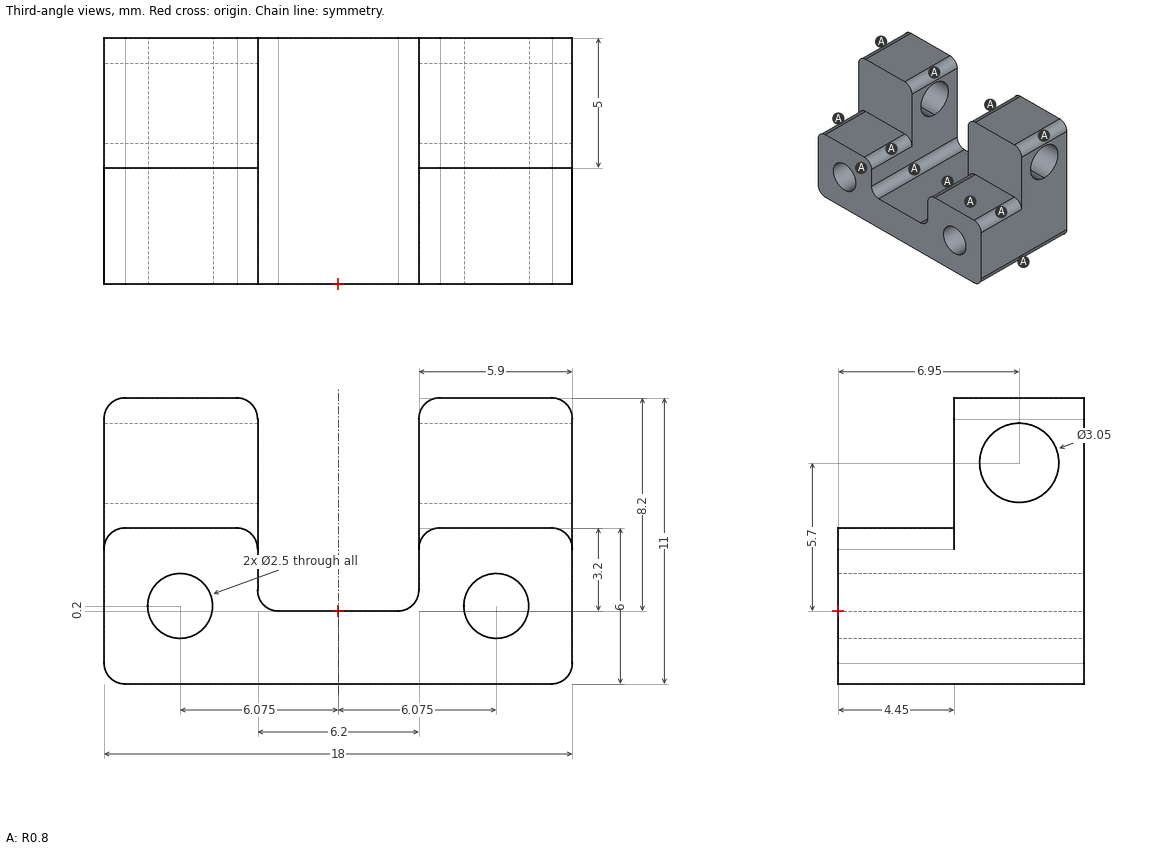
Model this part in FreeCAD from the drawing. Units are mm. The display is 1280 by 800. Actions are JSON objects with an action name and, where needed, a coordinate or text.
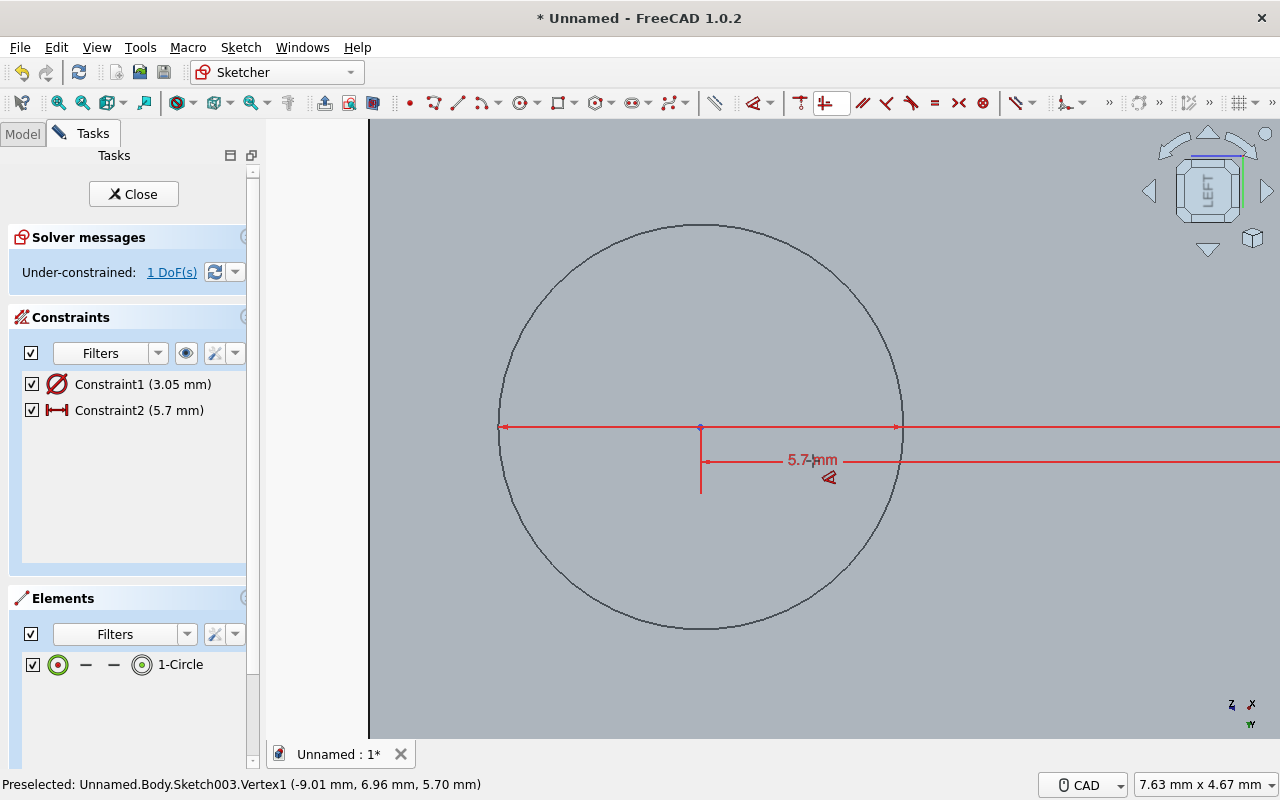
{"action": "left_click", "coordinate": [701, 427]}
{"action": "left_click", "coordinate": [667, 287]}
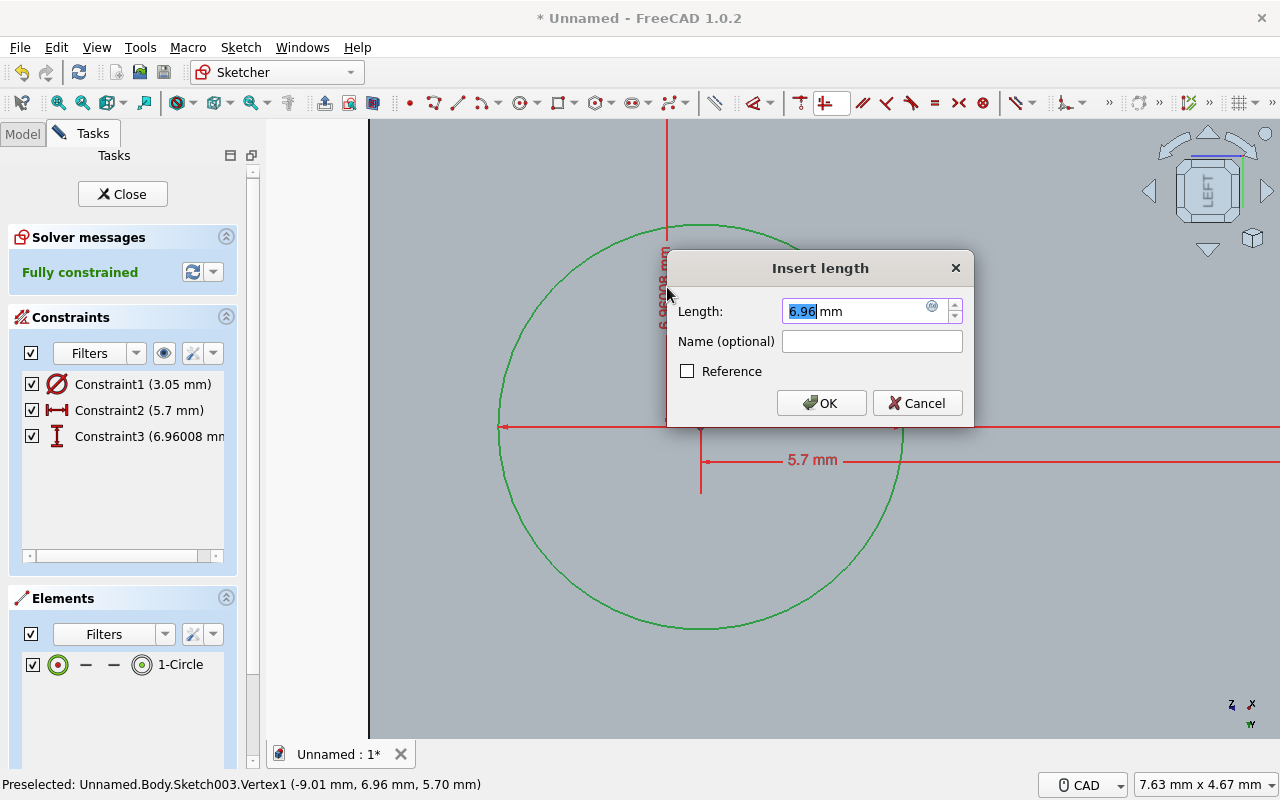
{"action": "type", "text": "6.95"}
{"action": "key", "text": "Return"}
{"action": "key", "text": "Escape"}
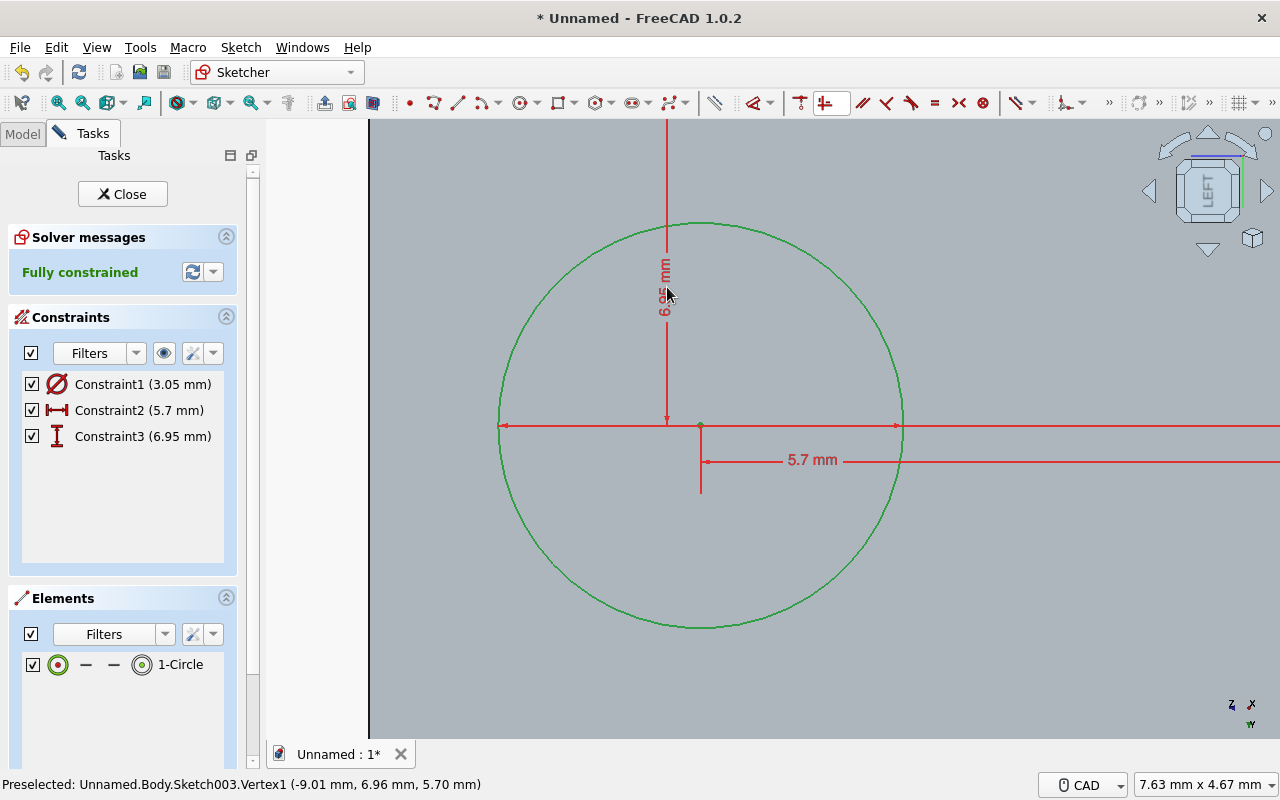
{"action": "left_click", "coordinate": [123, 194]}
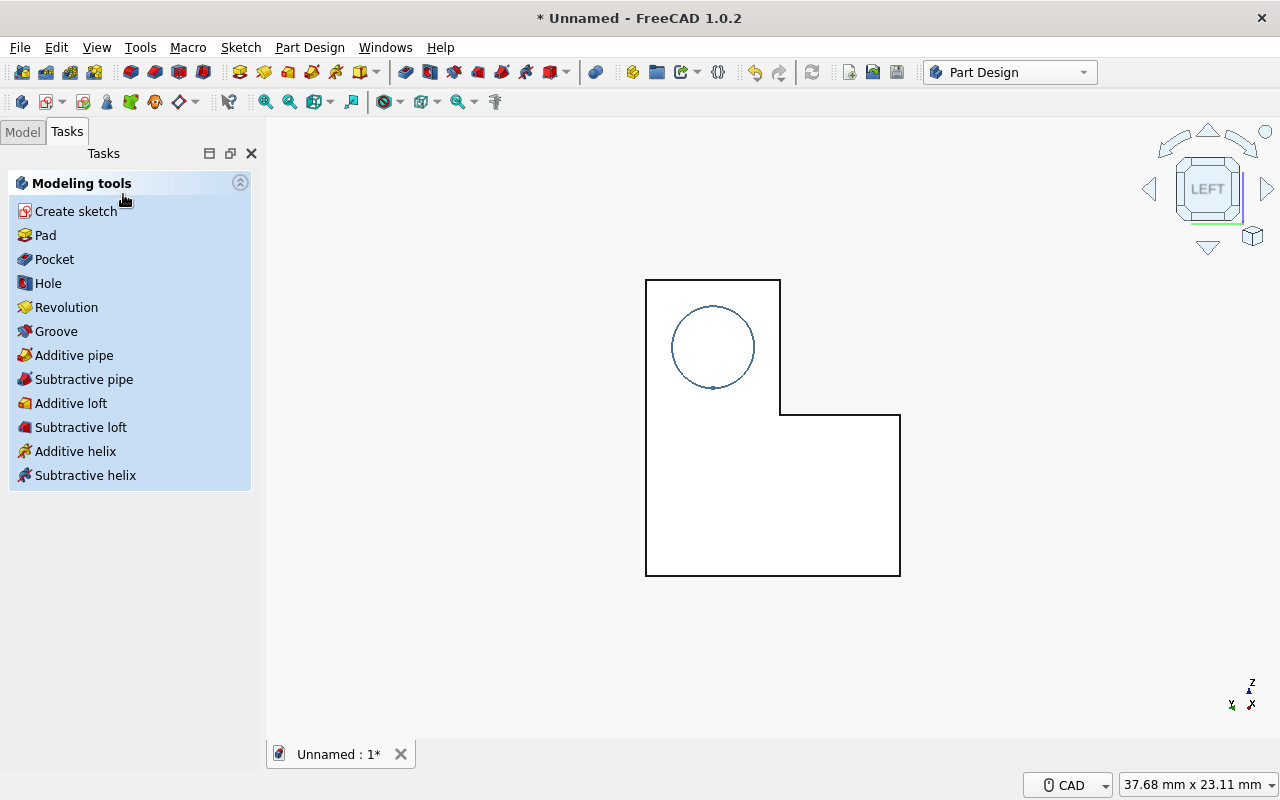
{"action": "left_click", "coordinate": [406, 72]}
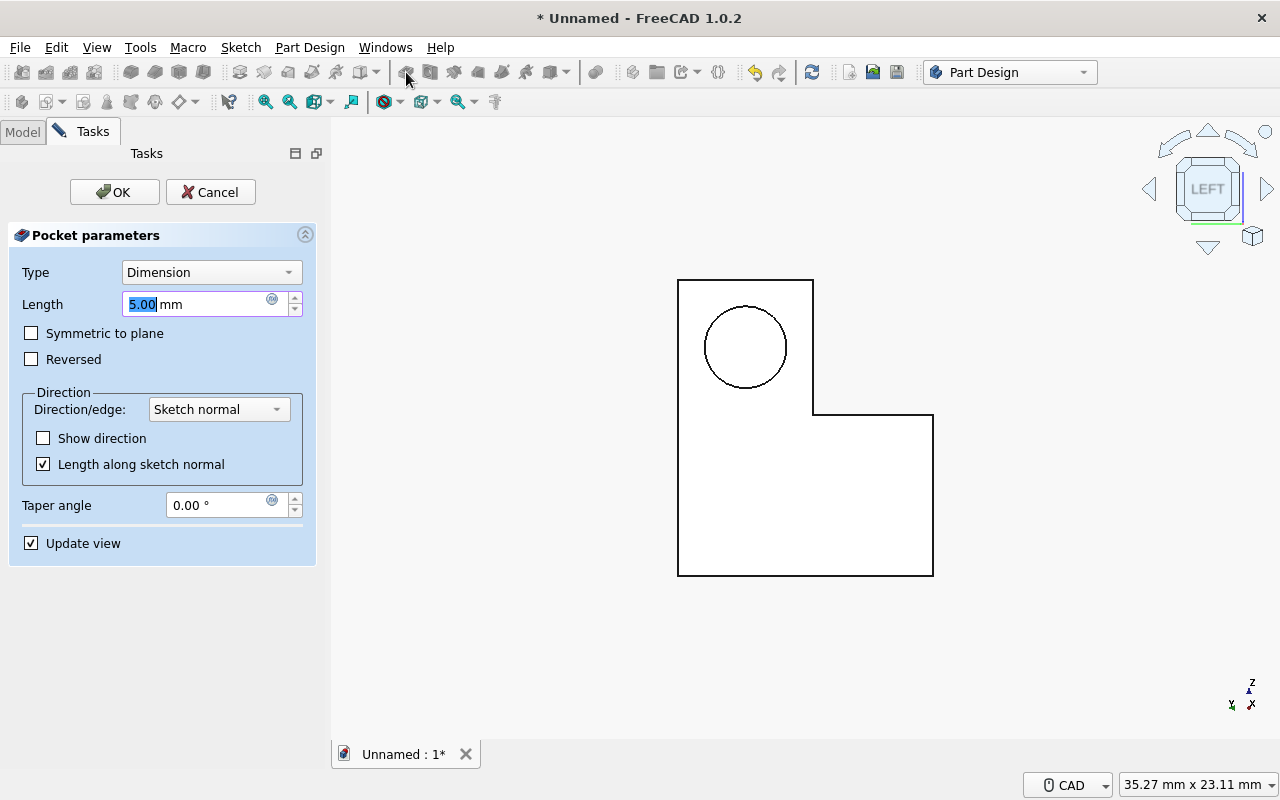
{"action": "left_click", "coordinate": [212, 272]}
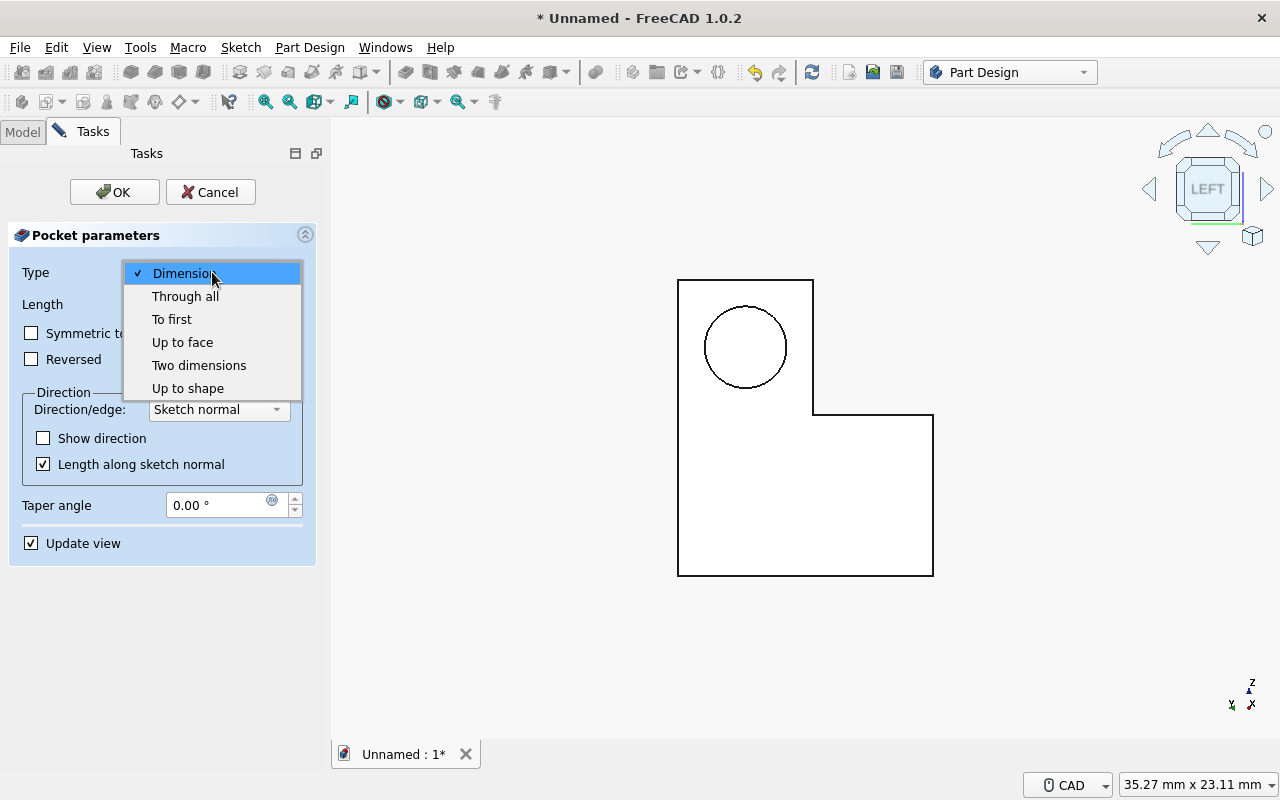
{"action": "left_click", "coordinate": [212, 296]}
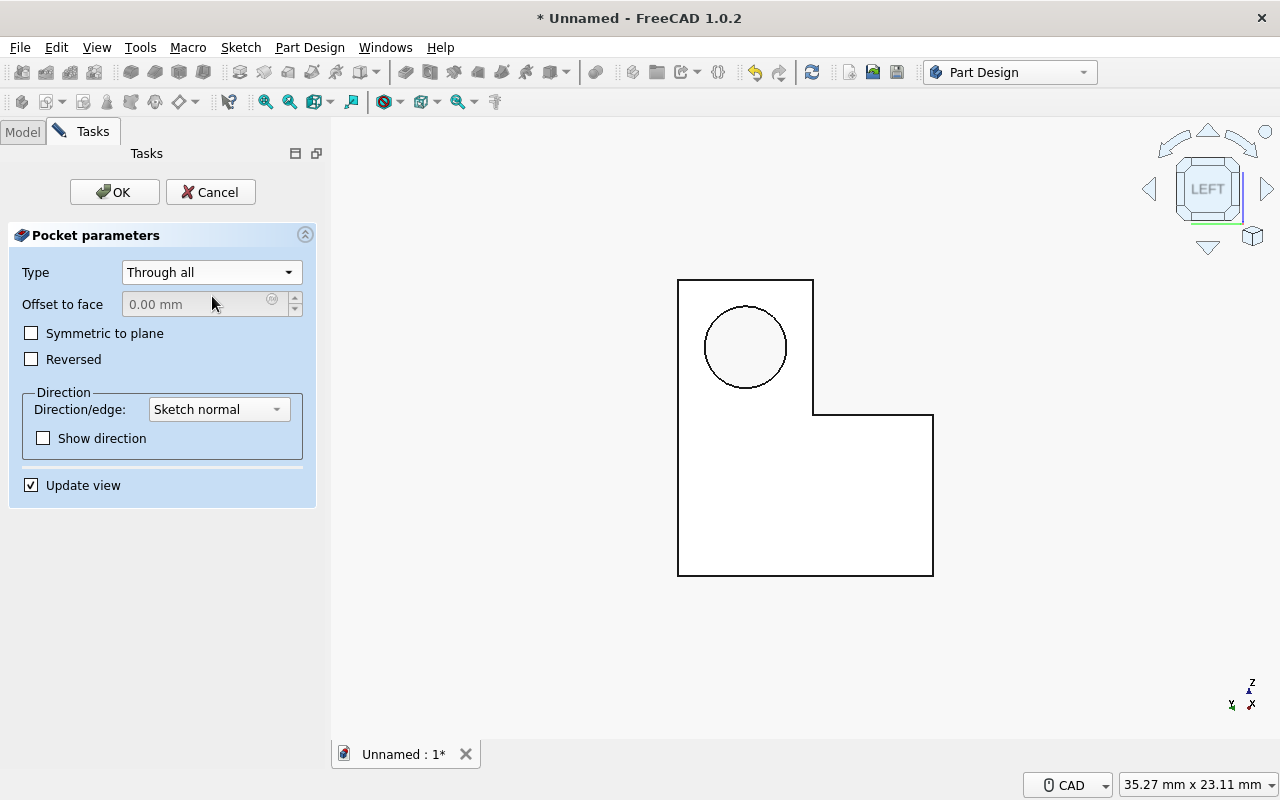
{"action": "left_click", "coordinate": [115, 192]}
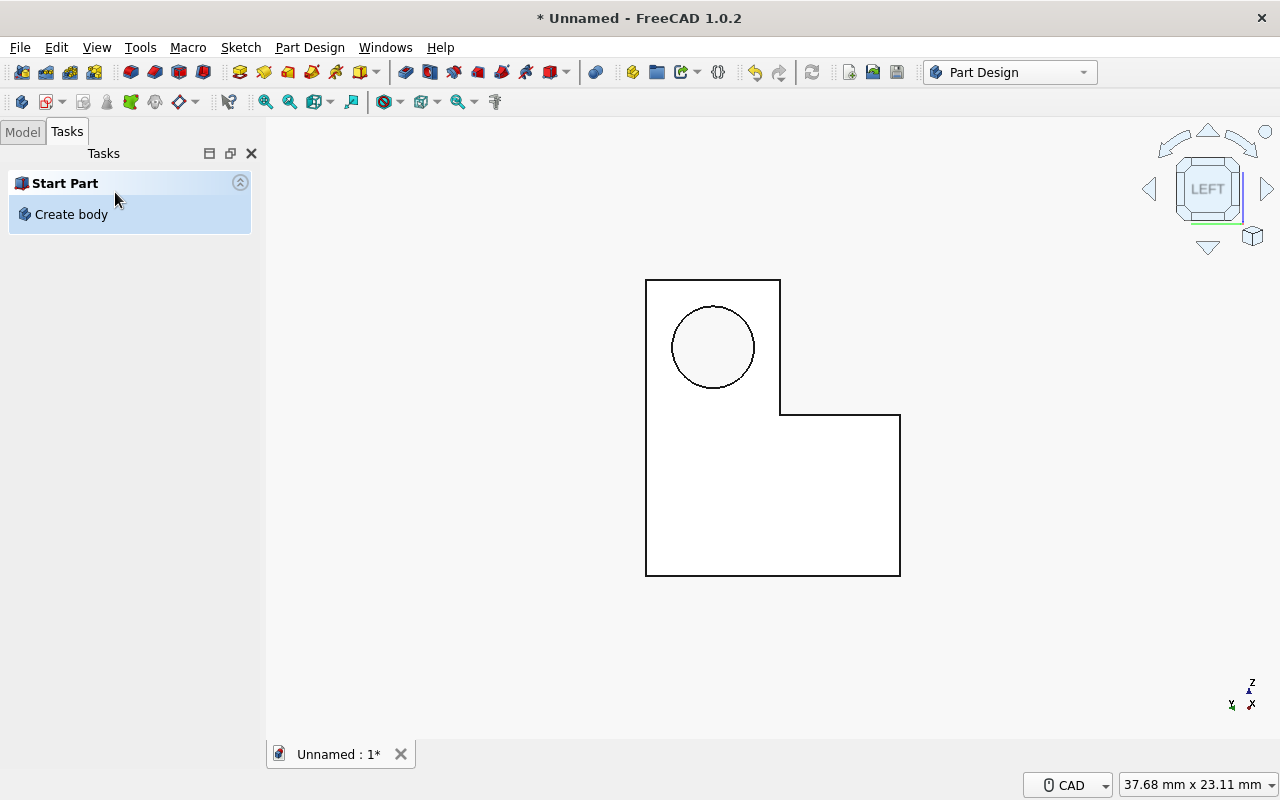
{"action": "left_click", "coordinate": [773, 575]}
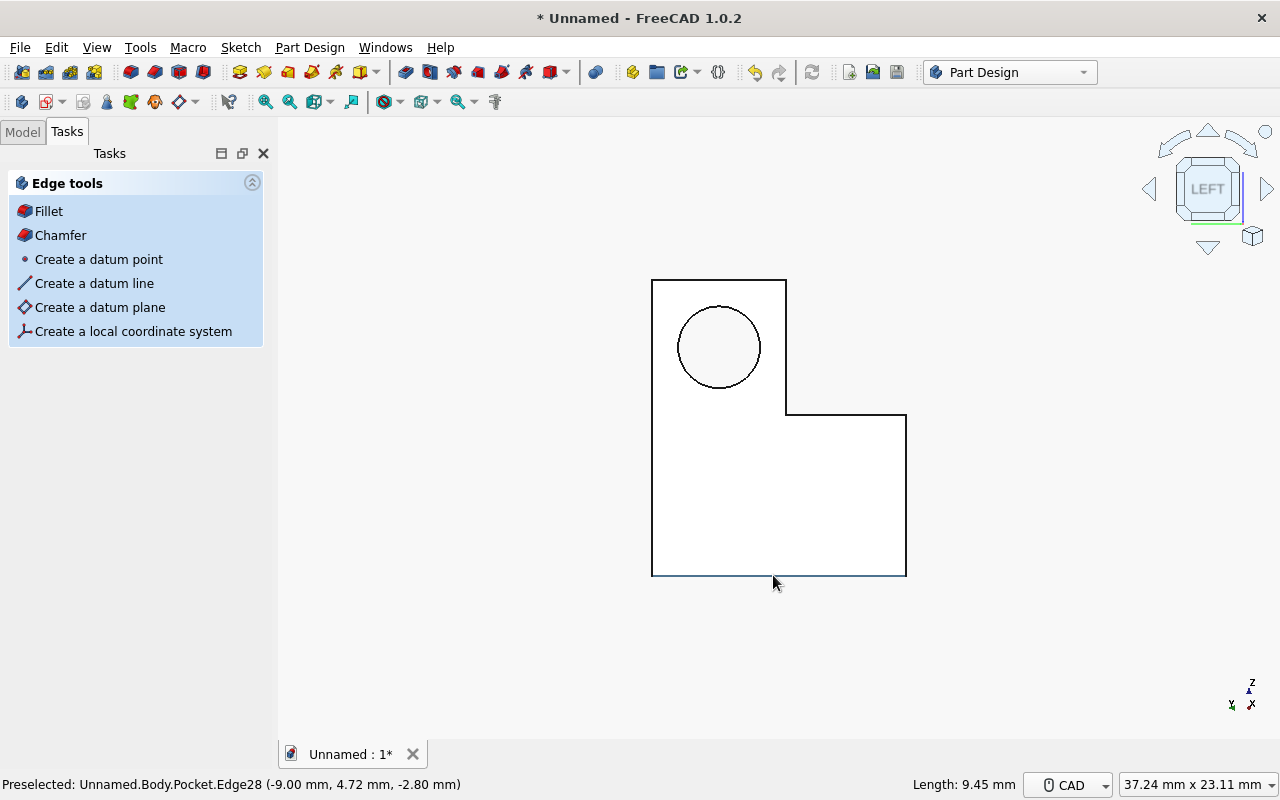
{"action": "left_click", "coordinate": [846, 414], "text": "ctrl"}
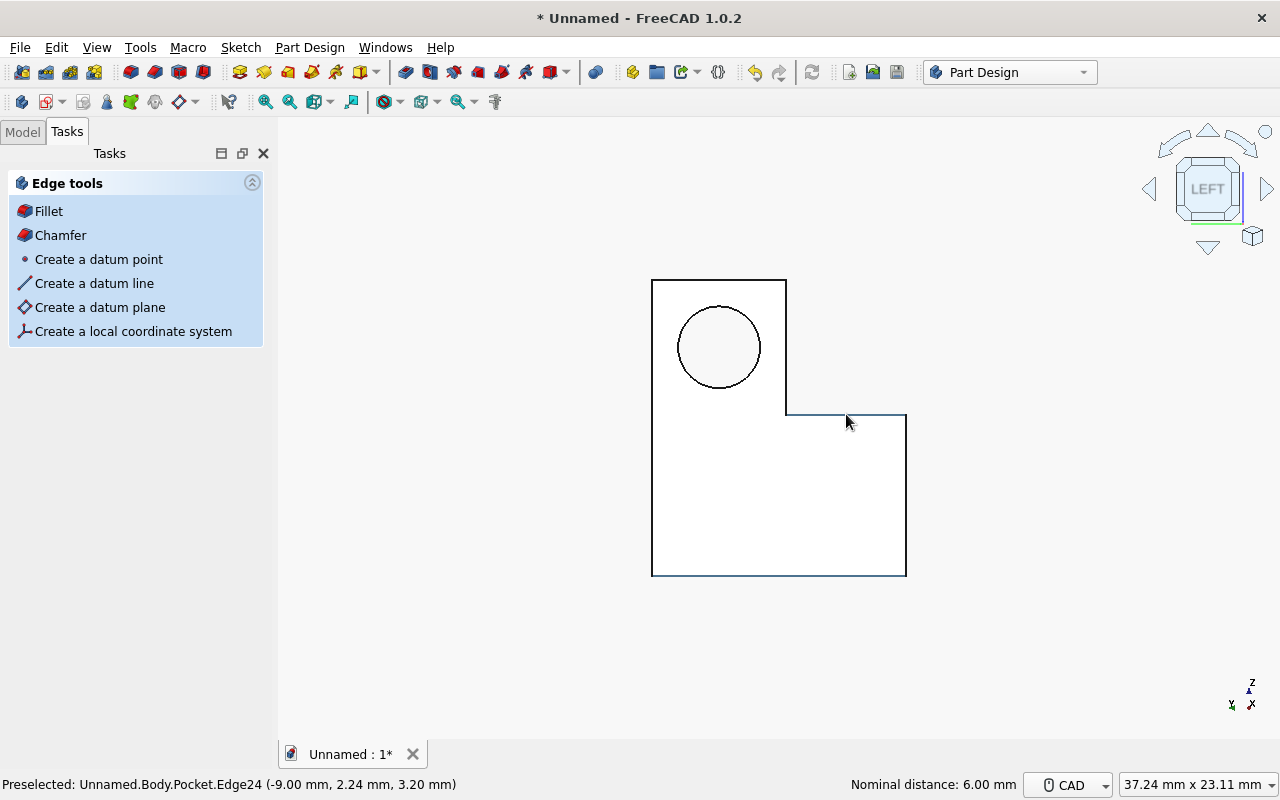
{"action": "left_click", "coordinate": [719, 279], "text": "ctrl"}